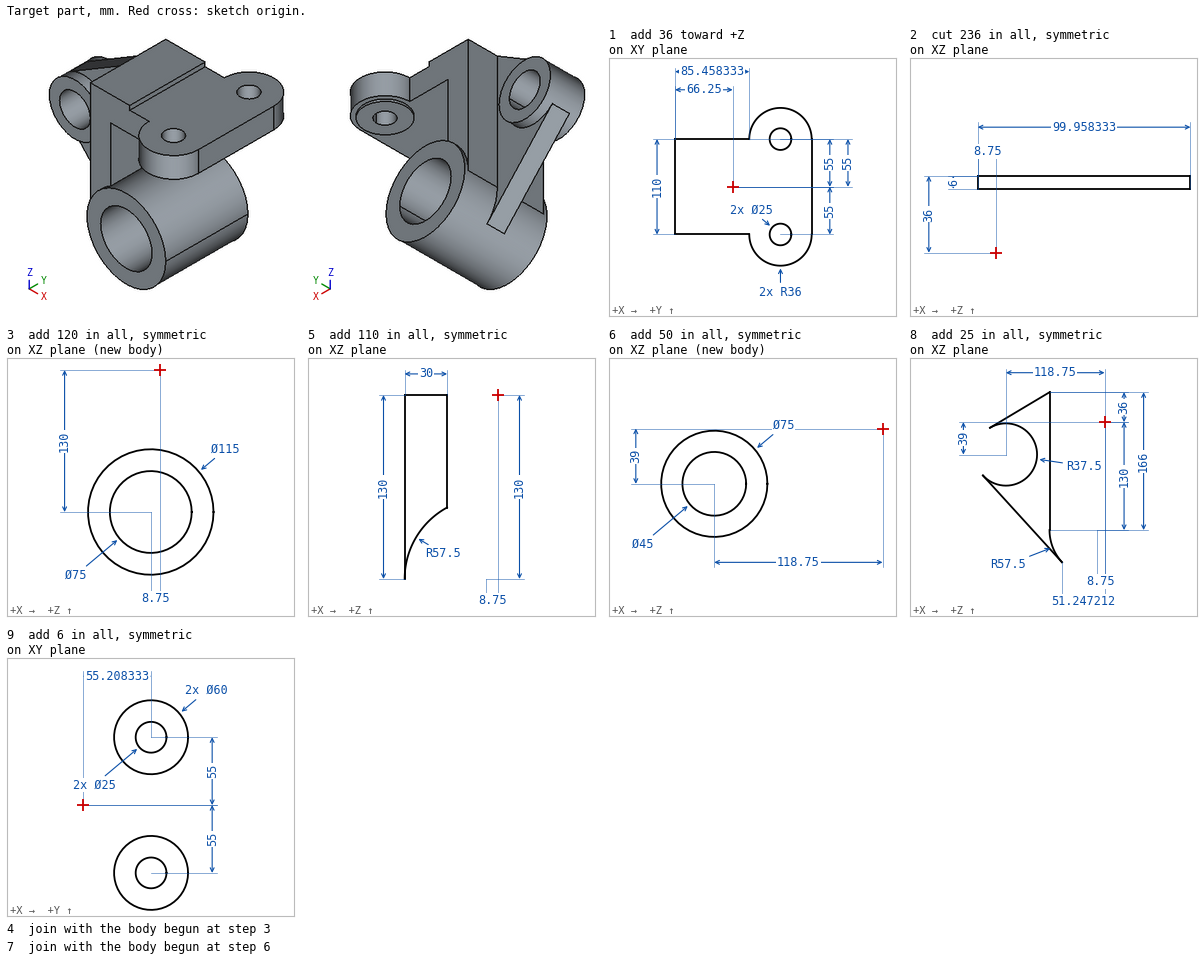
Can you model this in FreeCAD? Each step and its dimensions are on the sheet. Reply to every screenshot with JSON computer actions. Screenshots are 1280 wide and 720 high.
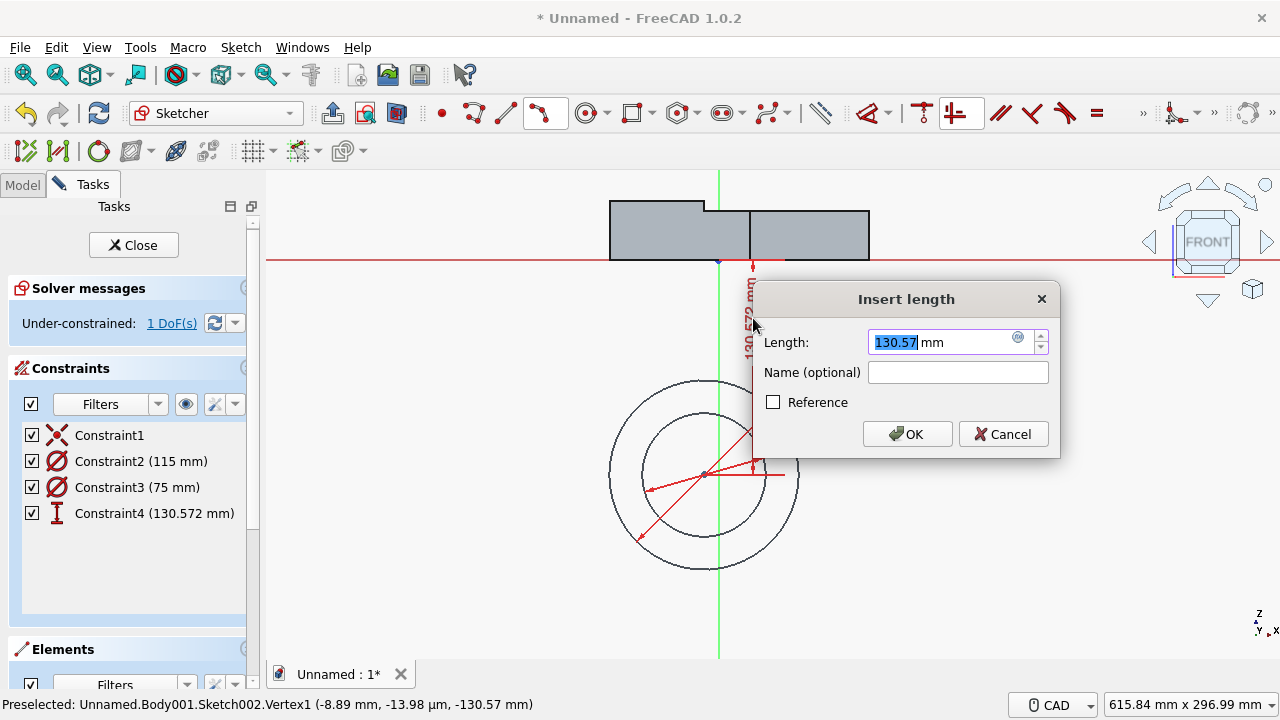
{"action": "type", "text": "130"}
{"action": "key", "text": "Return"}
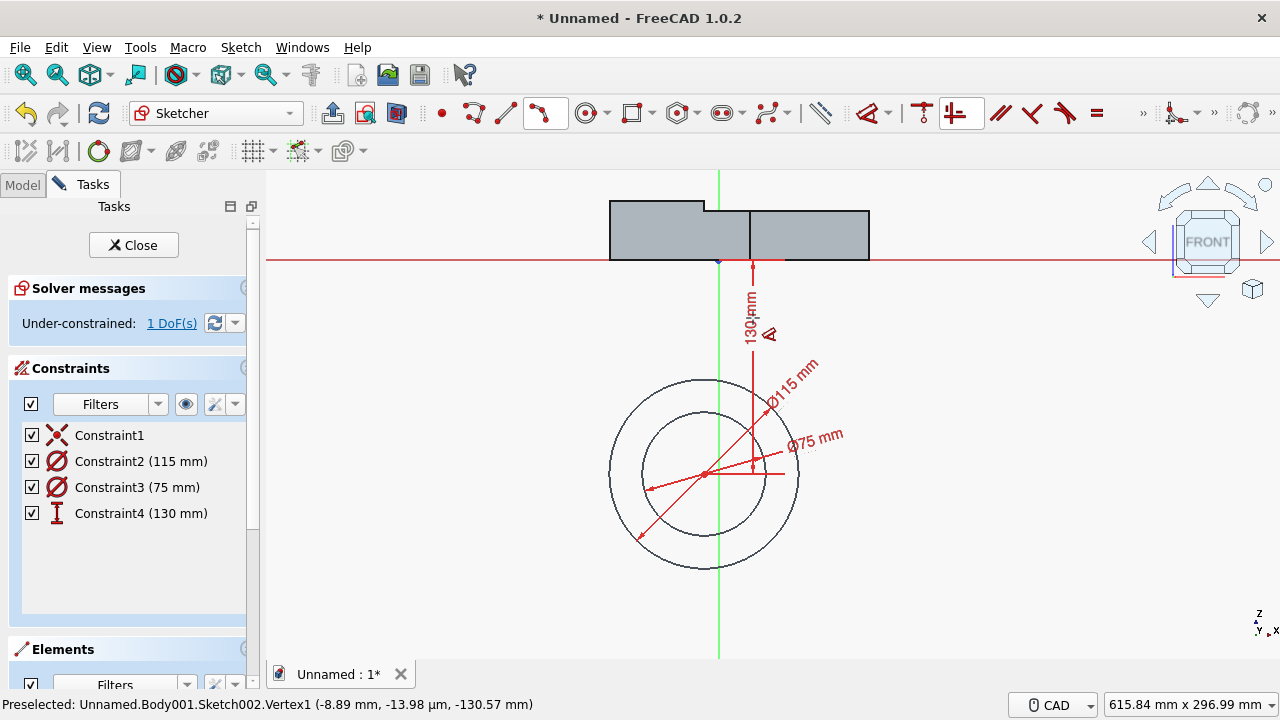
{"action": "scroll", "coordinate": [704, 474], "scroll_direction": "up", "scroll_amount": 6}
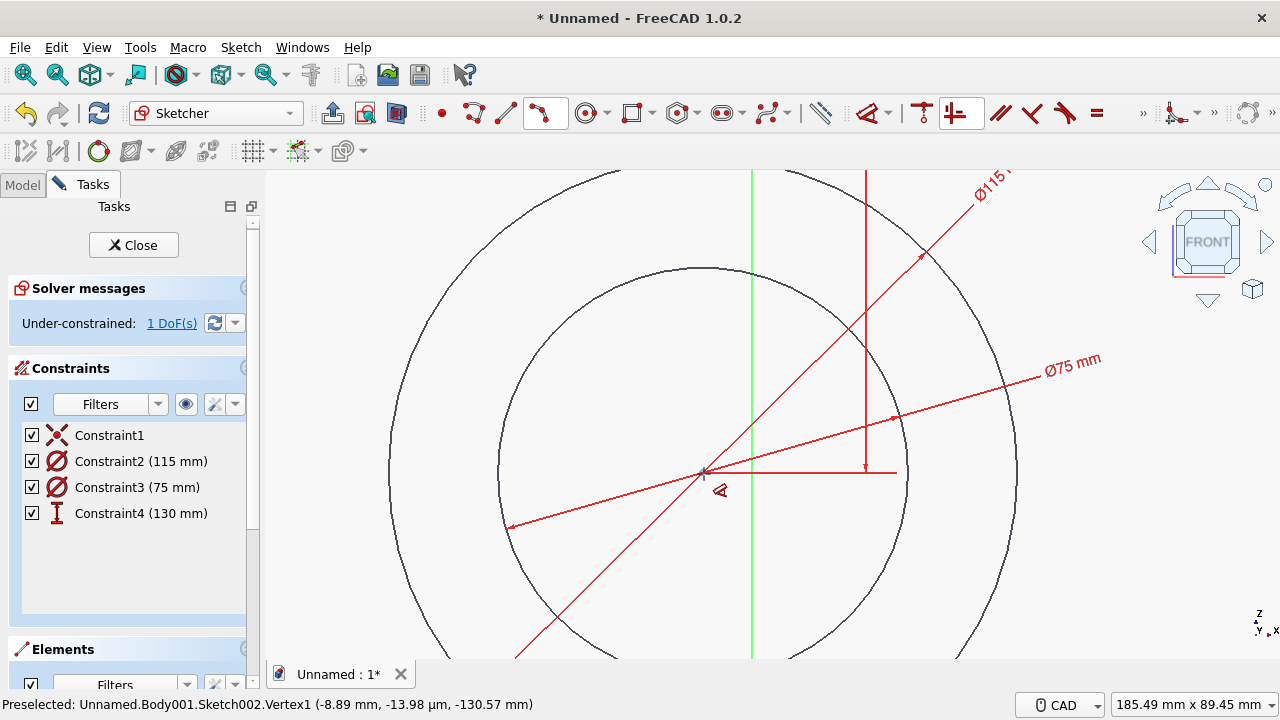
{"action": "left_click", "coordinate": [703, 473]}
{"action": "left_click", "coordinate": [727, 507]}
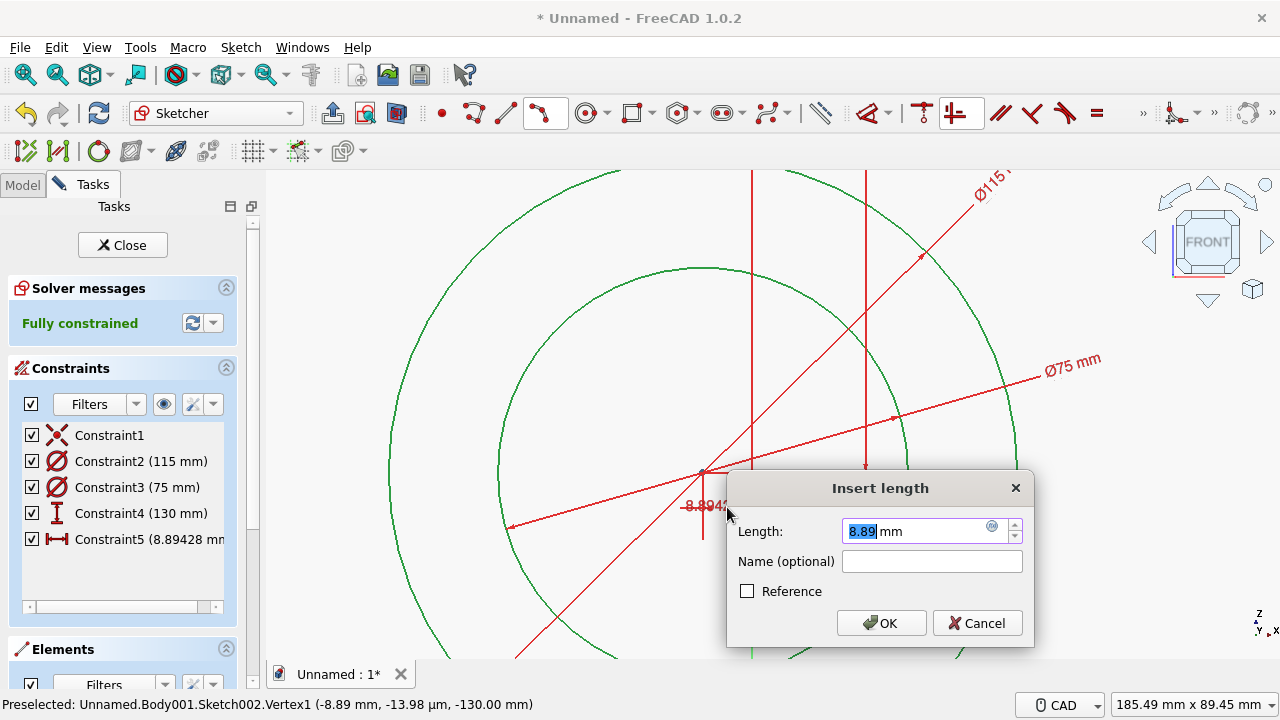
{"action": "type", "text": "8.75"}
{"action": "key", "text": "Return"}
{"action": "key", "text": "Escape"}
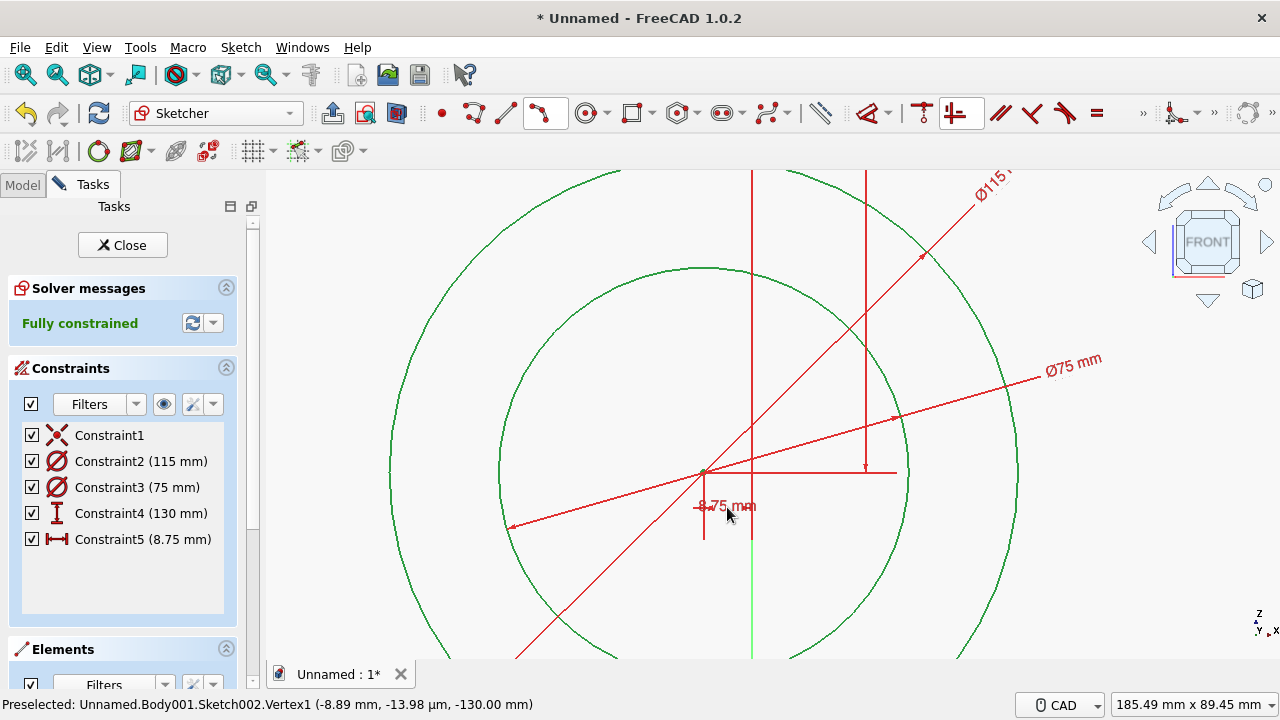
{"action": "left_click", "coordinate": [123, 245]}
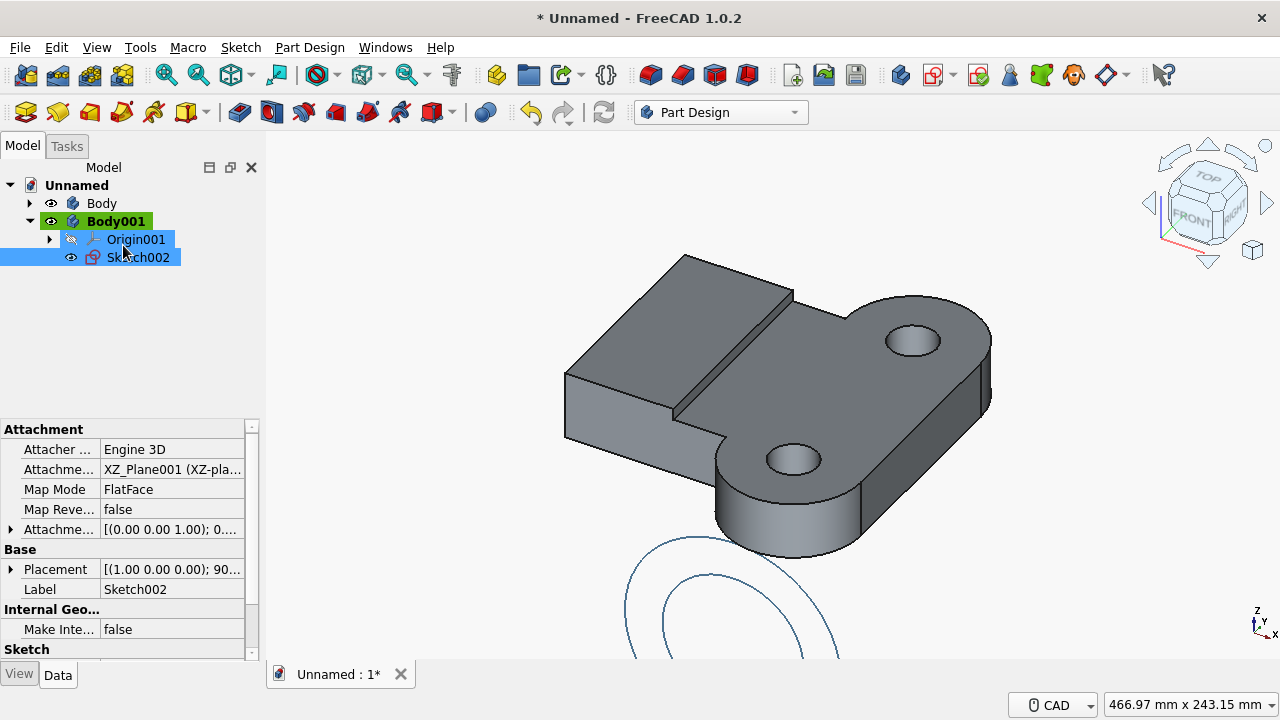
{"action": "left_click", "coordinate": [26, 112]}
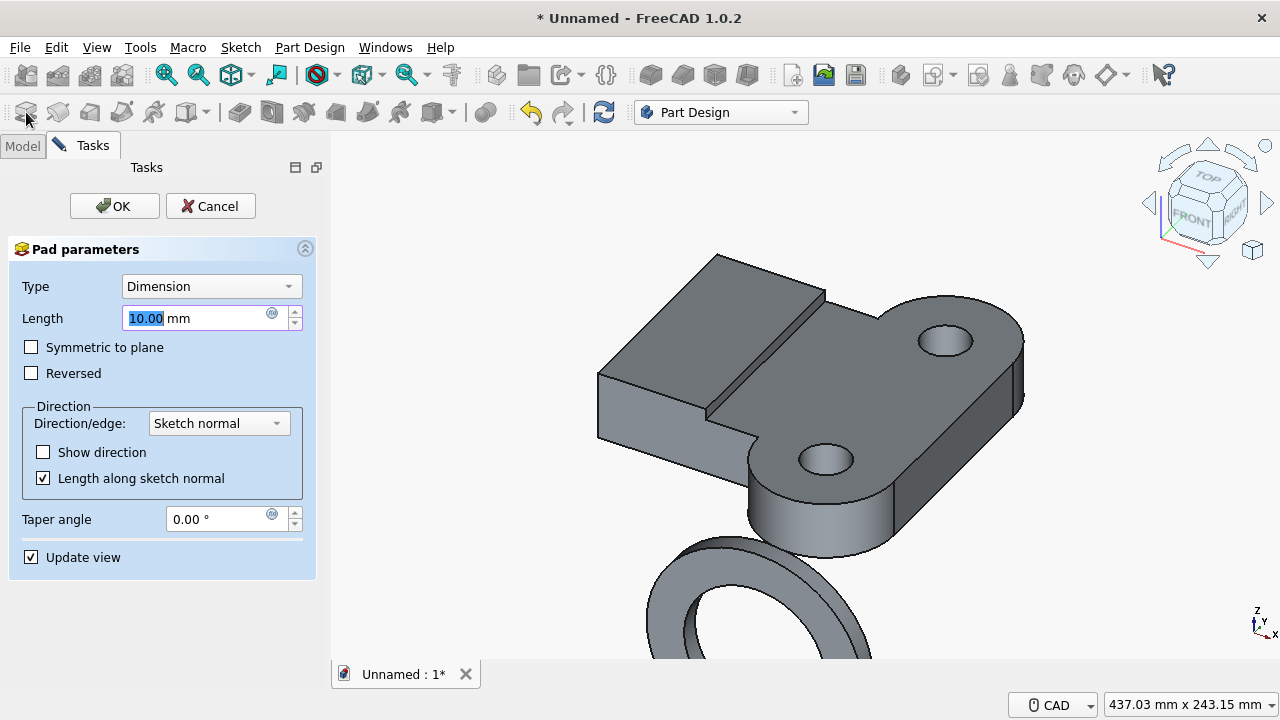
{"action": "type", "text": "120"}
{"action": "key", "text": "Tab"}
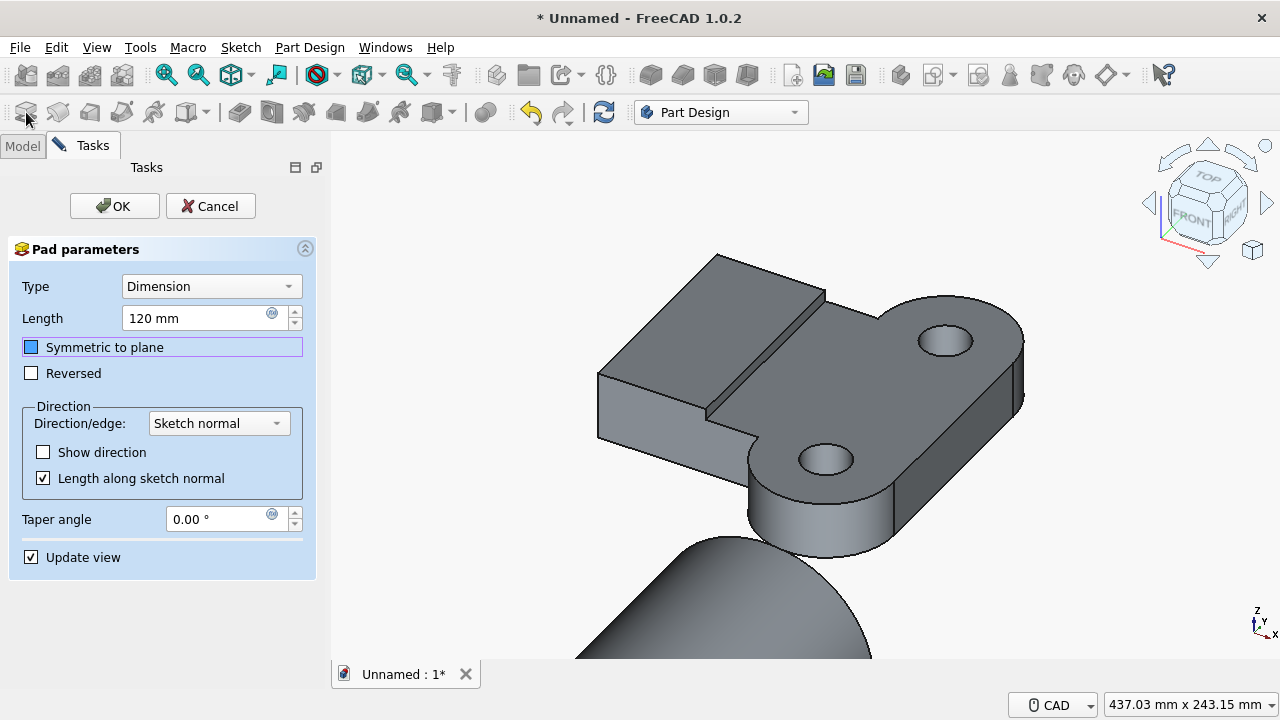
{"action": "left_click", "coordinate": [30, 347]}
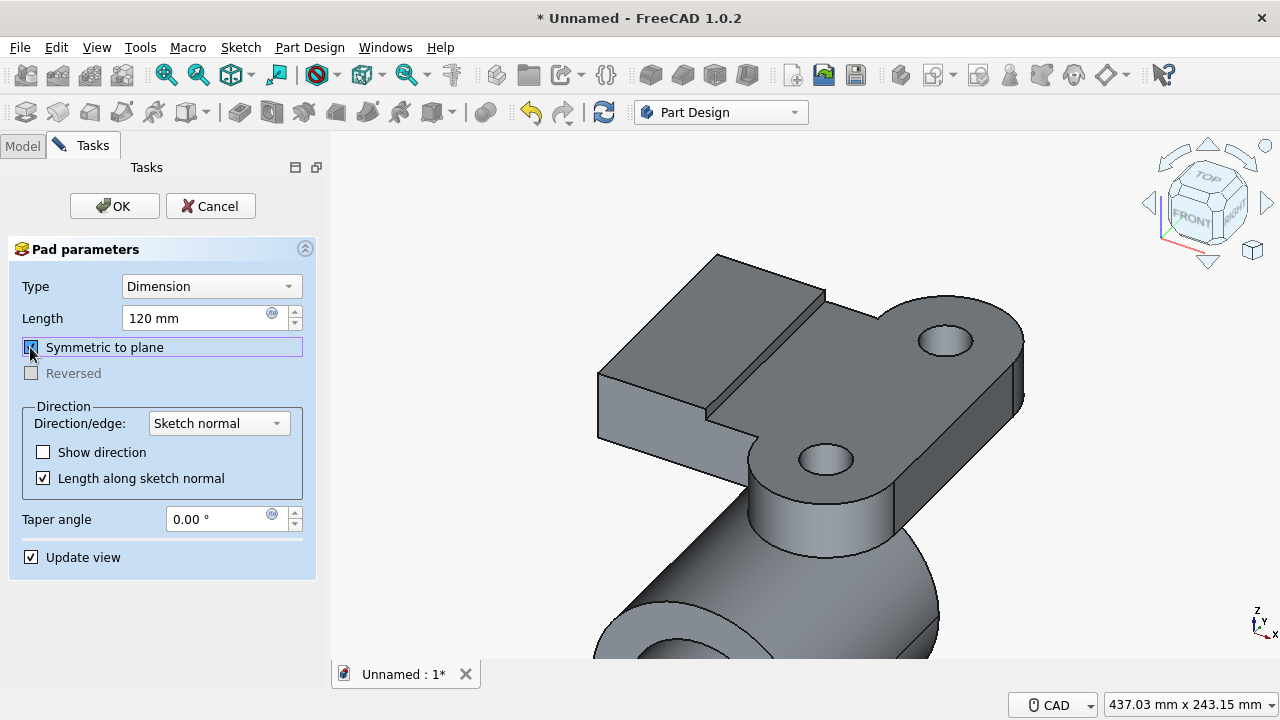
{"action": "left_click", "coordinate": [115, 206]}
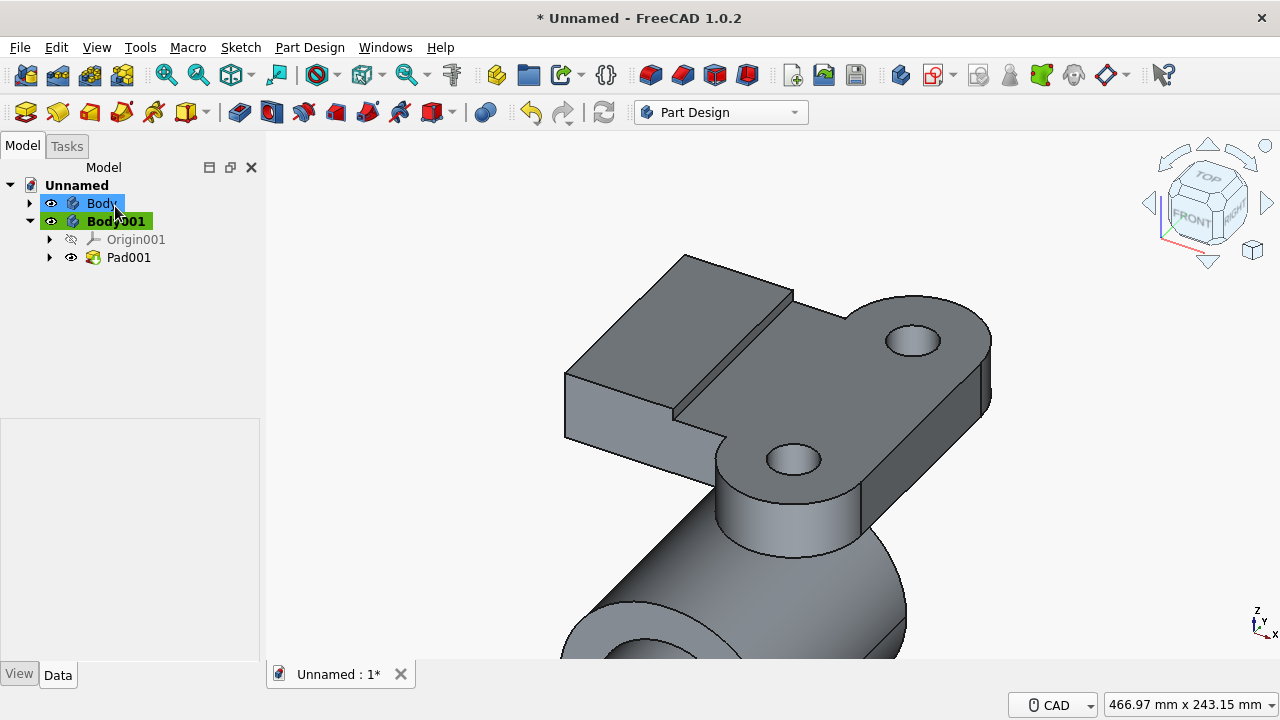
{"action": "left_click", "coordinate": [168, 76]}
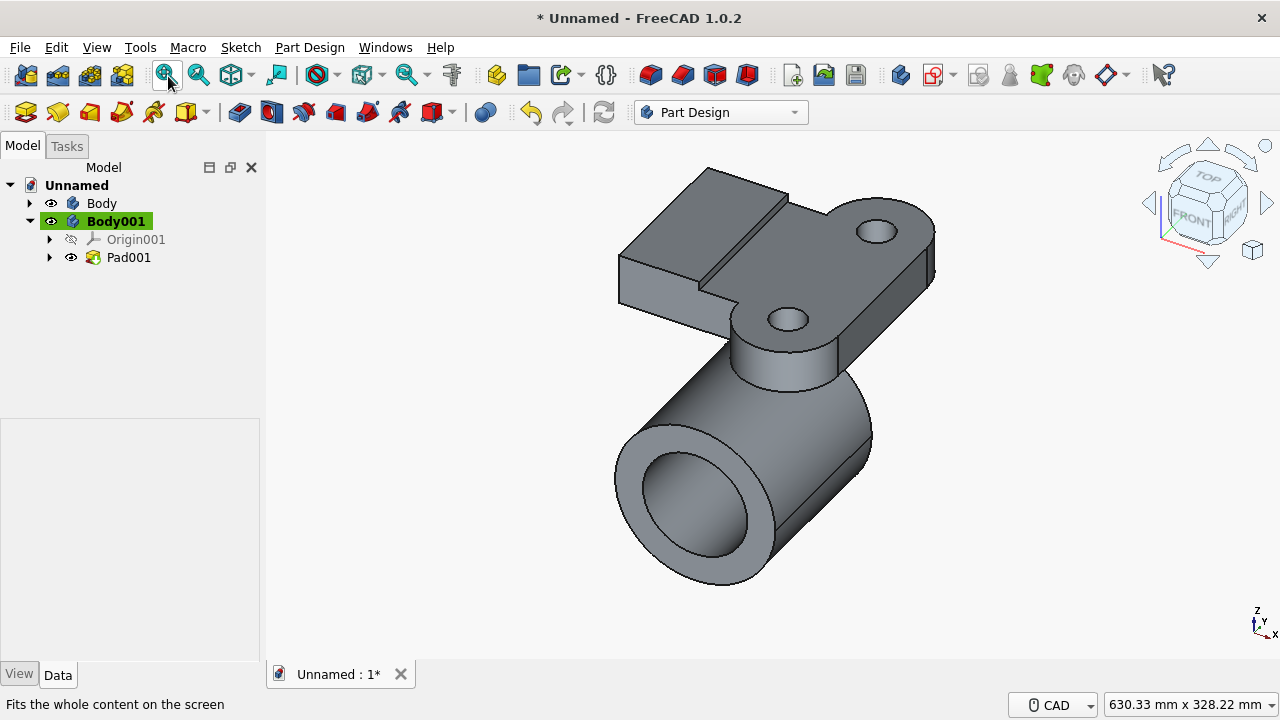
{"action": "double_click", "coordinate": [96, 203]}